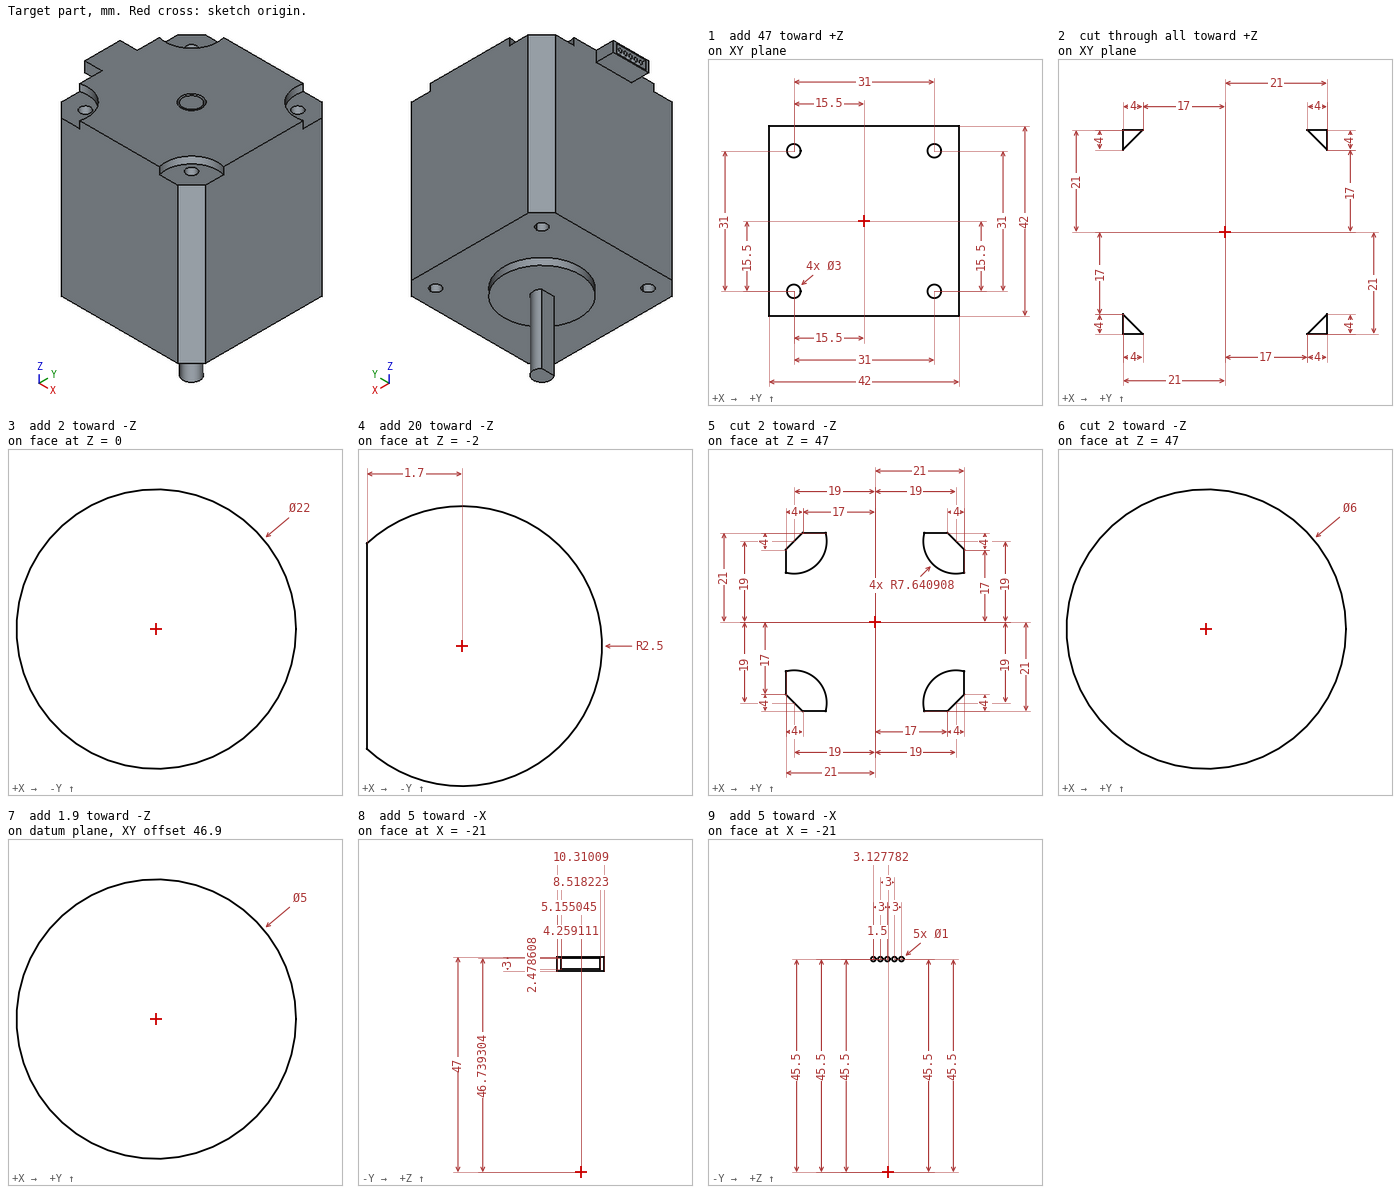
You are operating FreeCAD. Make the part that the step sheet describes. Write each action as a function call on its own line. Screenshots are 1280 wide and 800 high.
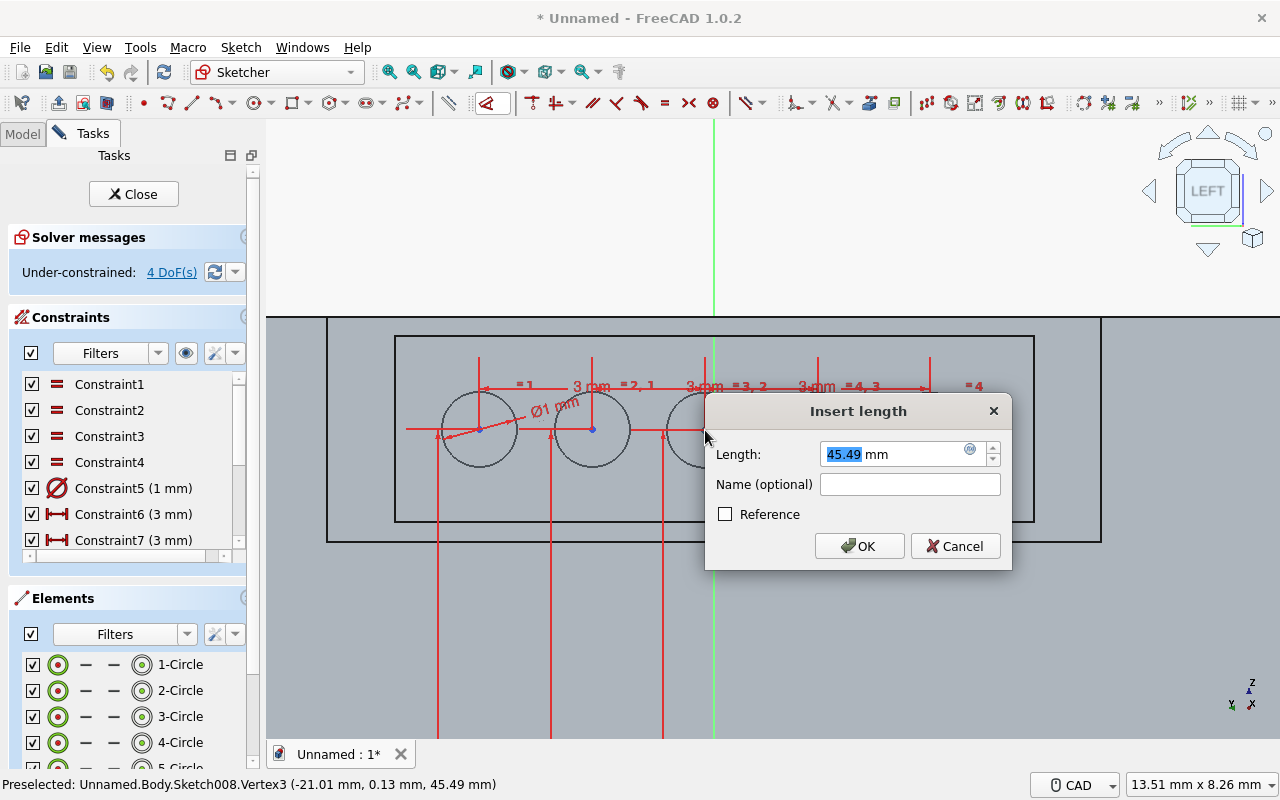
text(45.5)
key(Return)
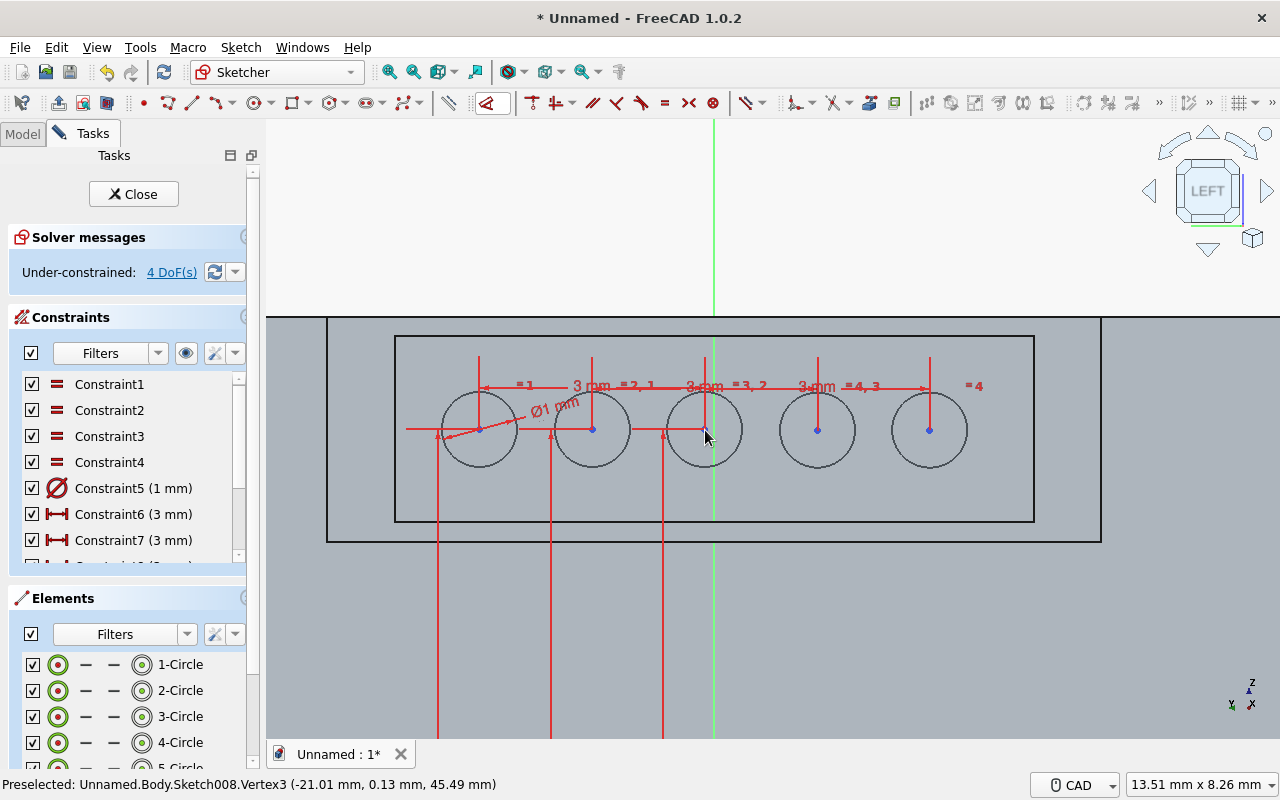
click(818, 430)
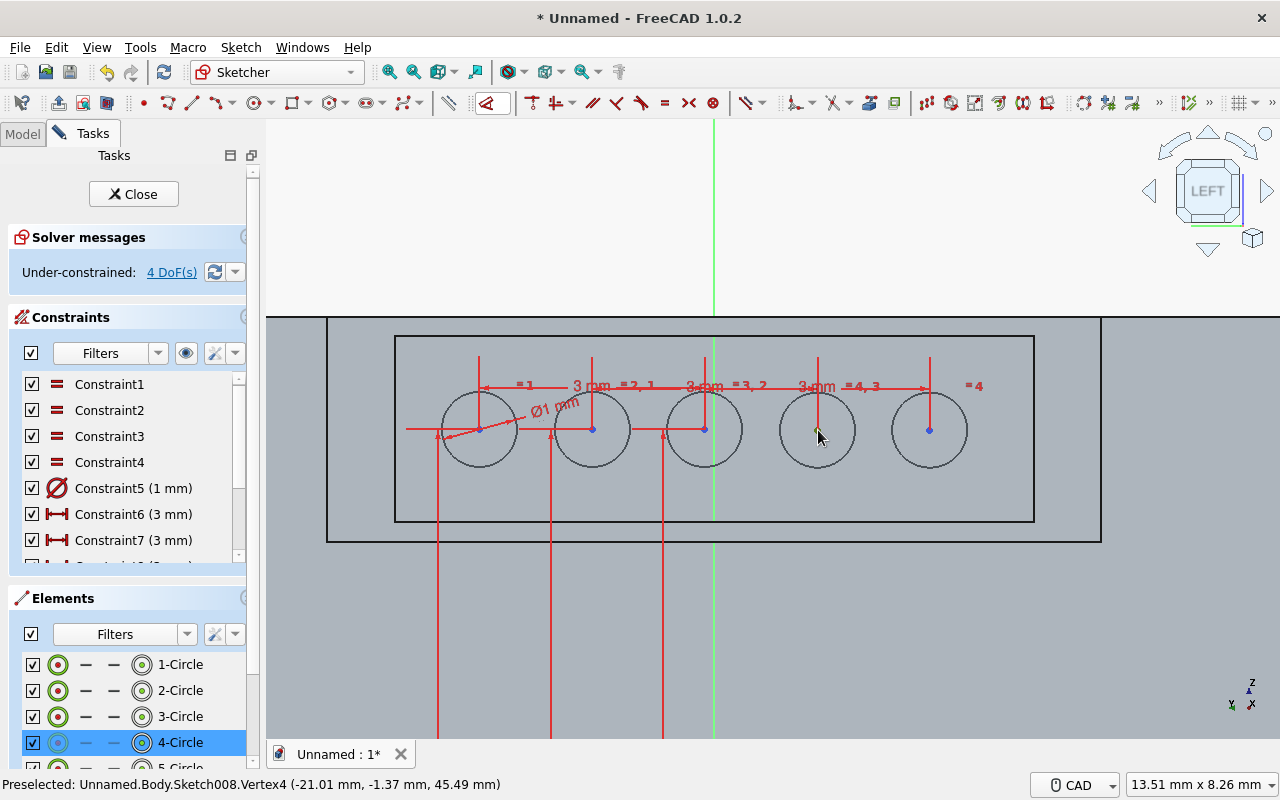
key(i)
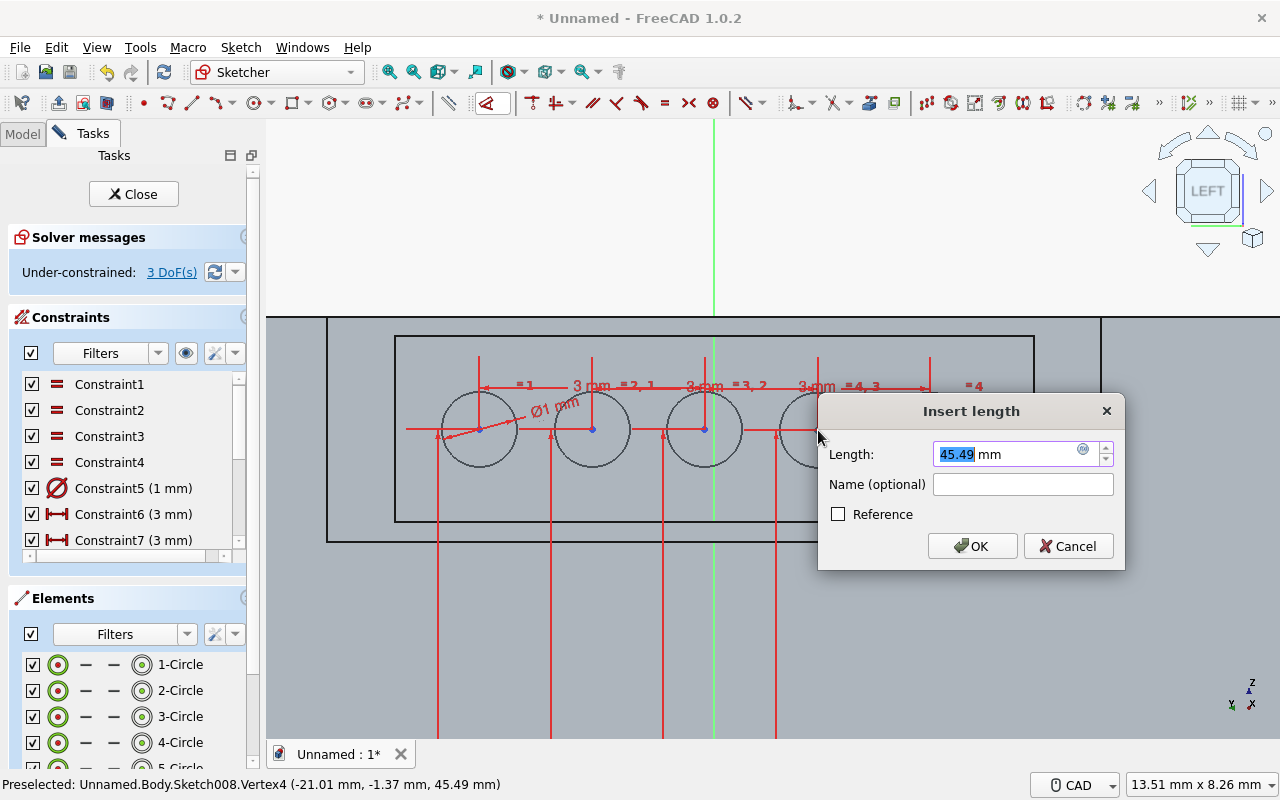
text(45.5)
key(Return)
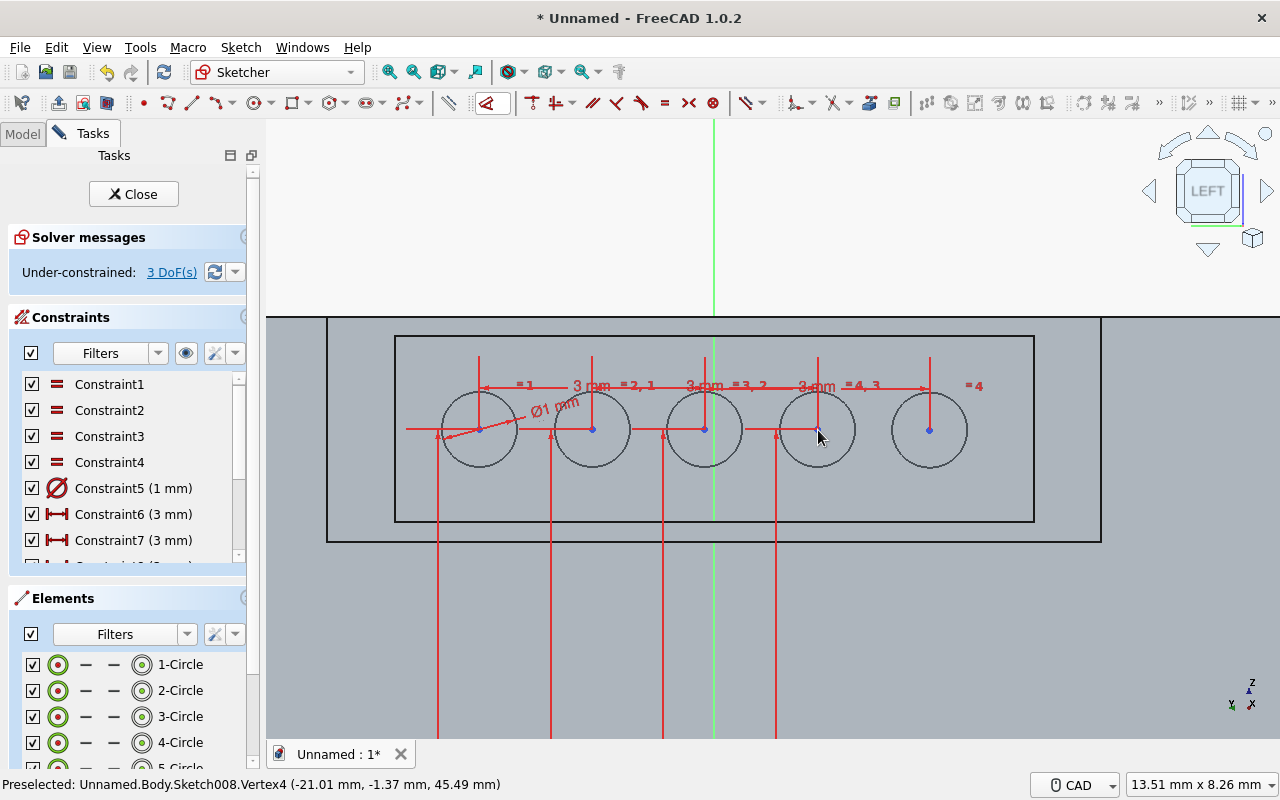
click(930, 430)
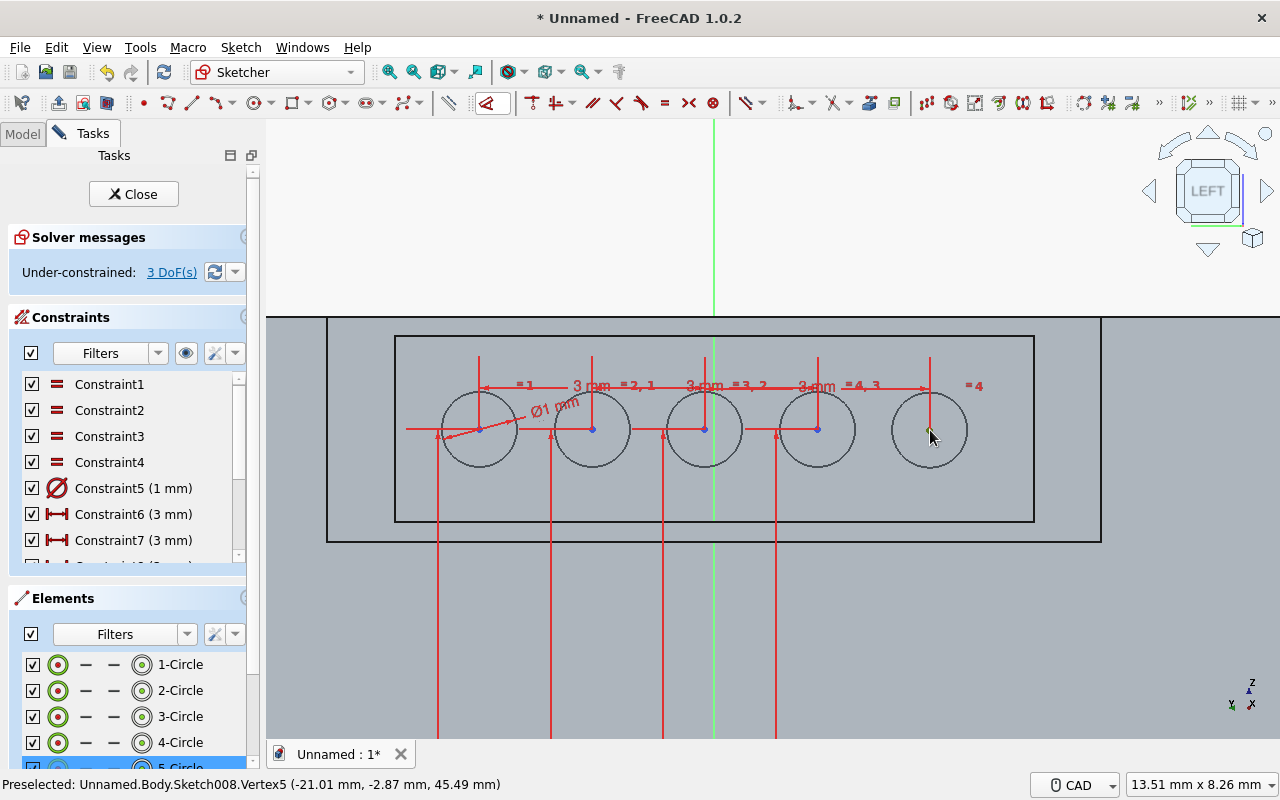
key(i)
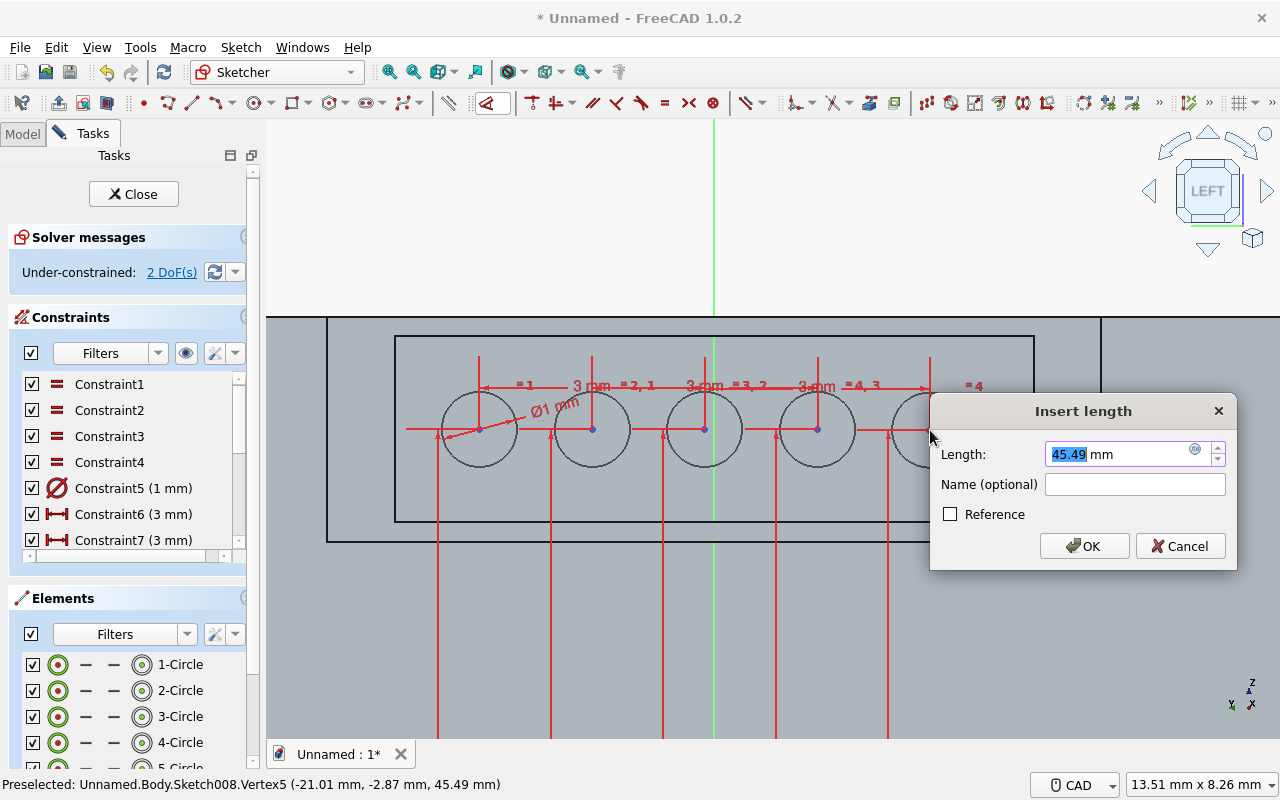
text(45.5)
key(Return)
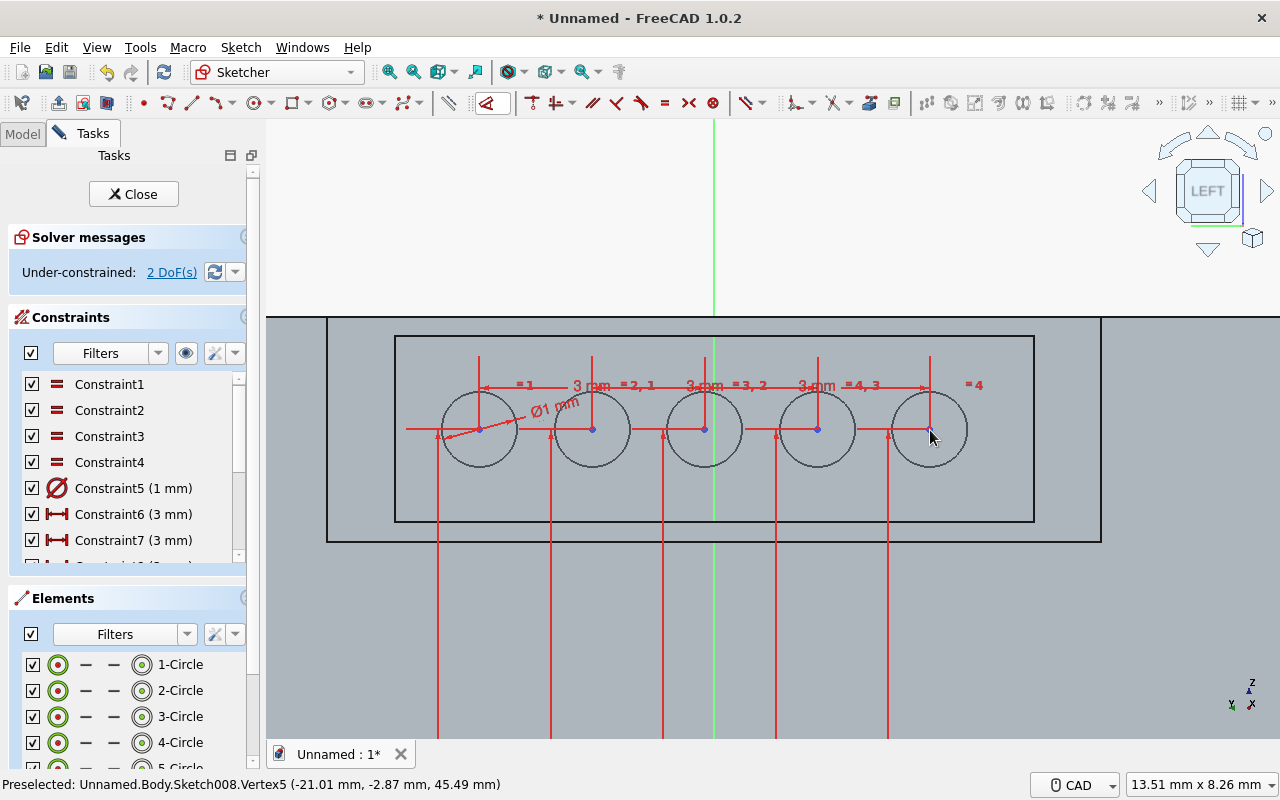
click(479, 429)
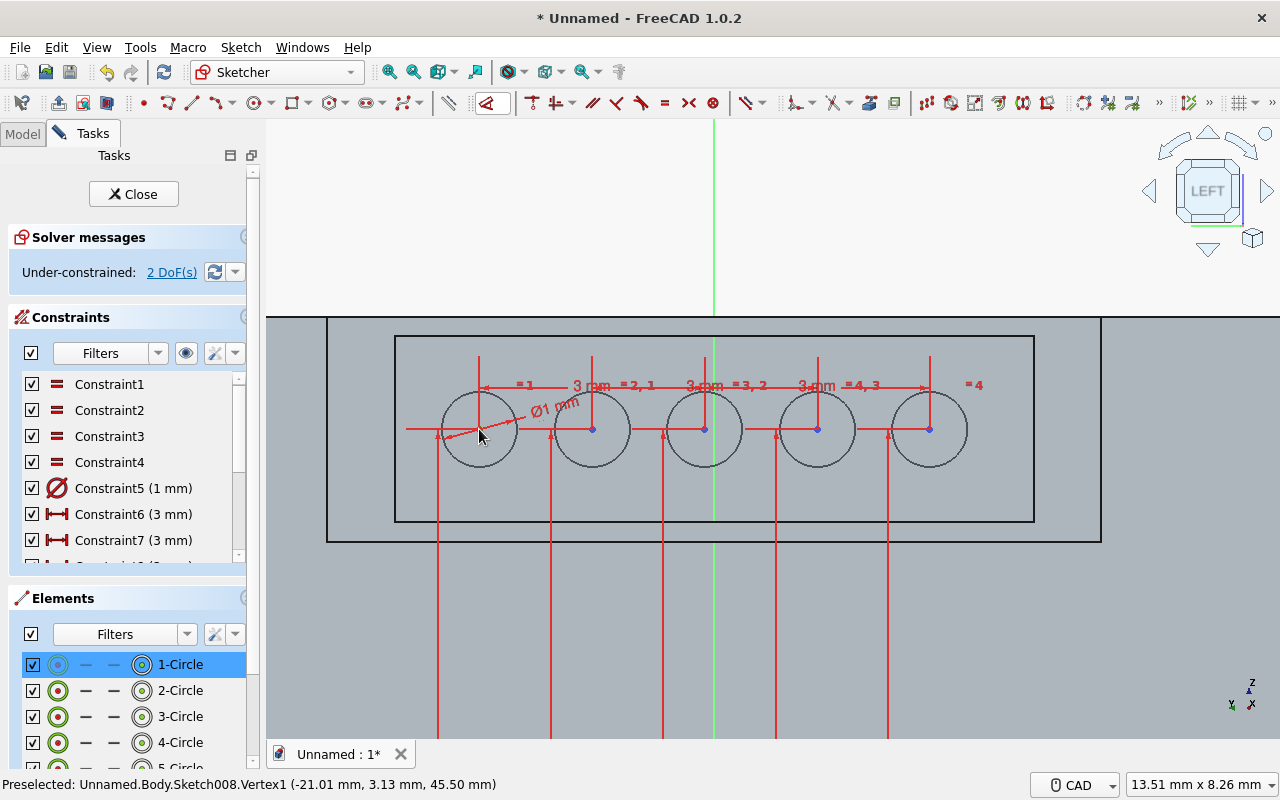
click(592, 429)